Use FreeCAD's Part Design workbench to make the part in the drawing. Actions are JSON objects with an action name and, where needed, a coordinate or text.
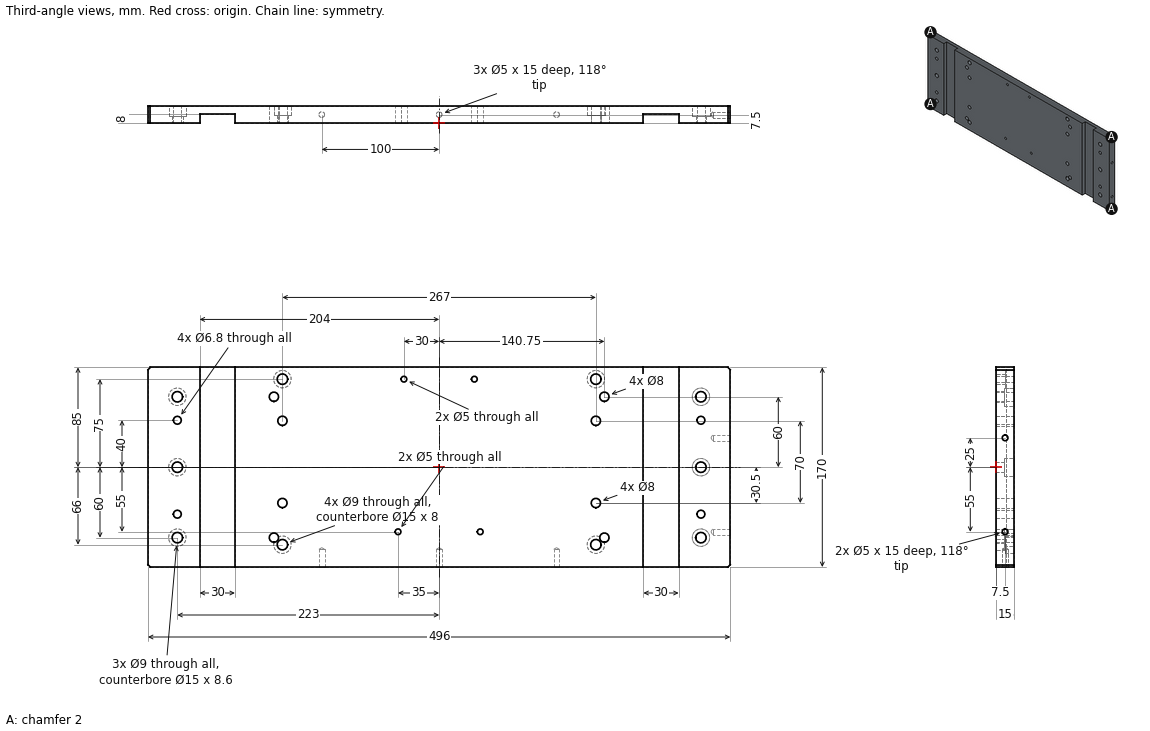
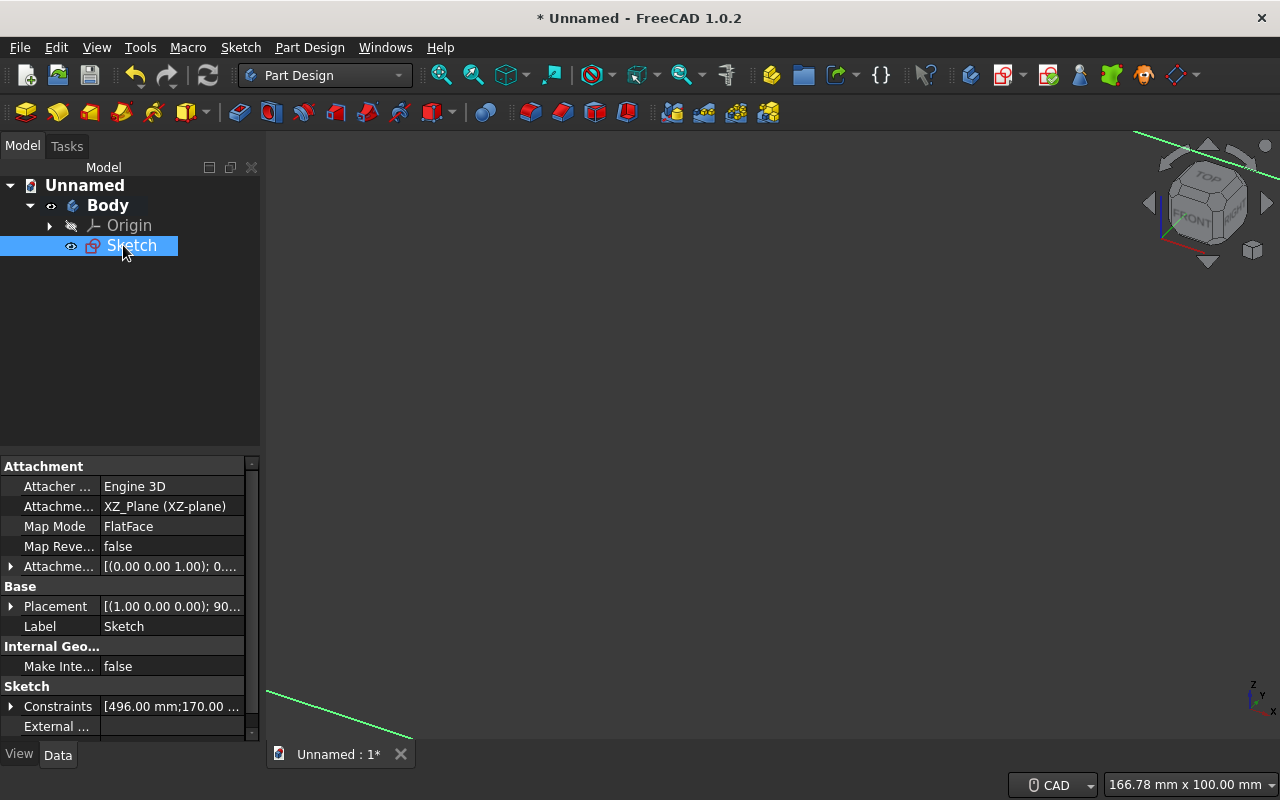
{"action": "left_click", "coordinate": [26, 112]}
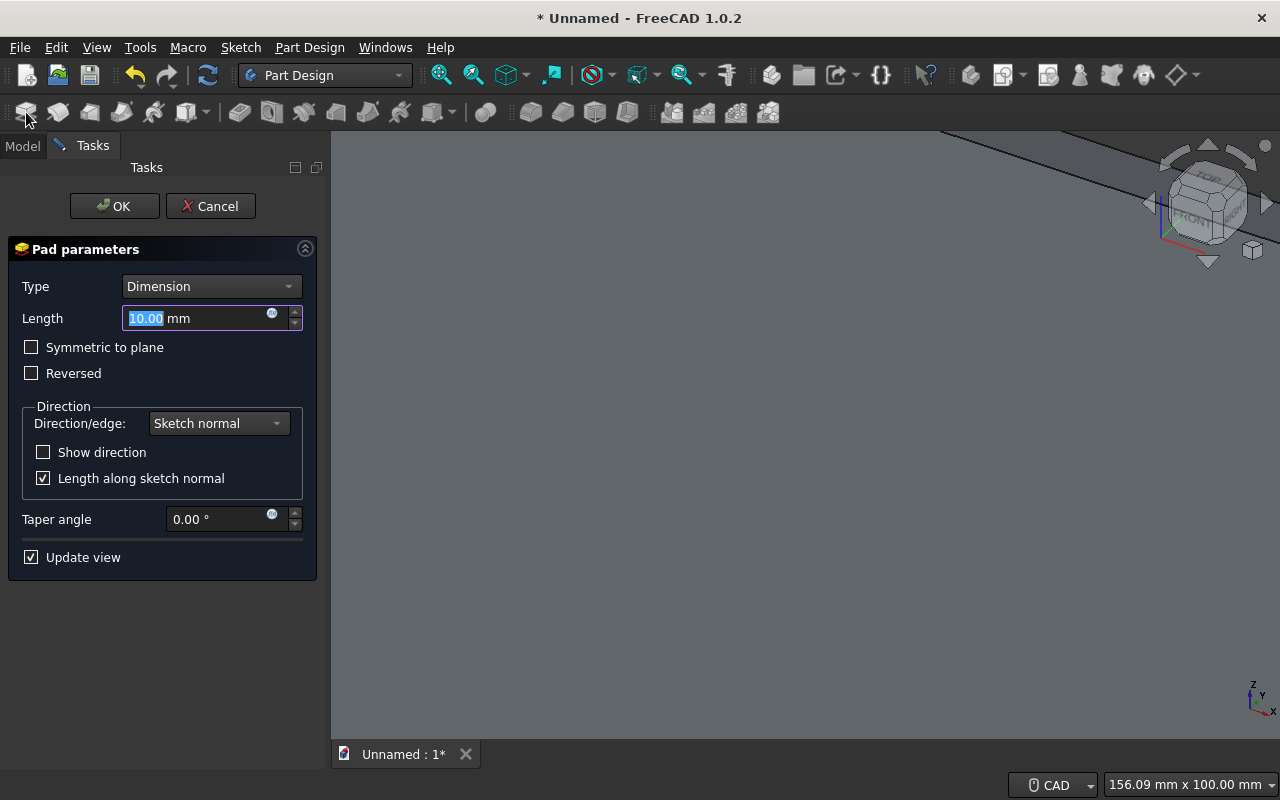
{"action": "type", "text": "15"}
{"action": "key", "text": "Tab"}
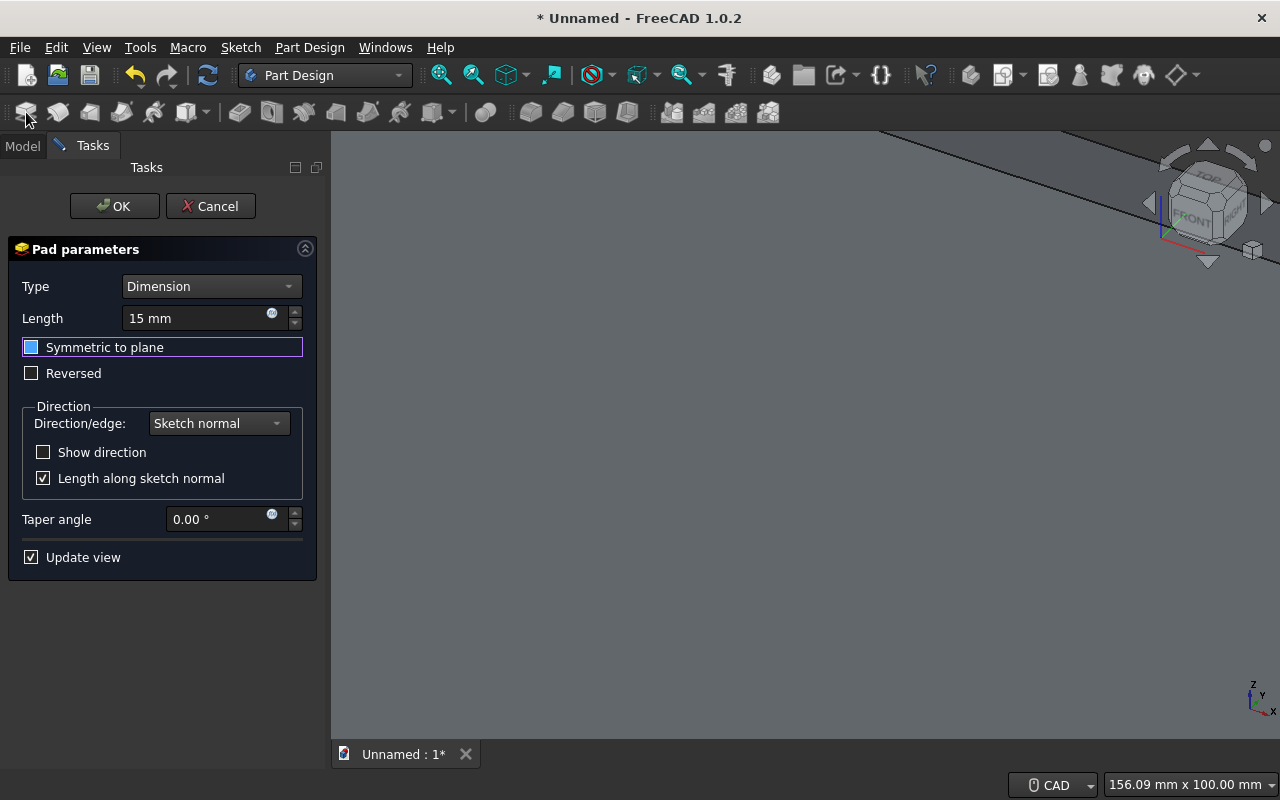
{"action": "left_click", "coordinate": [30, 373]}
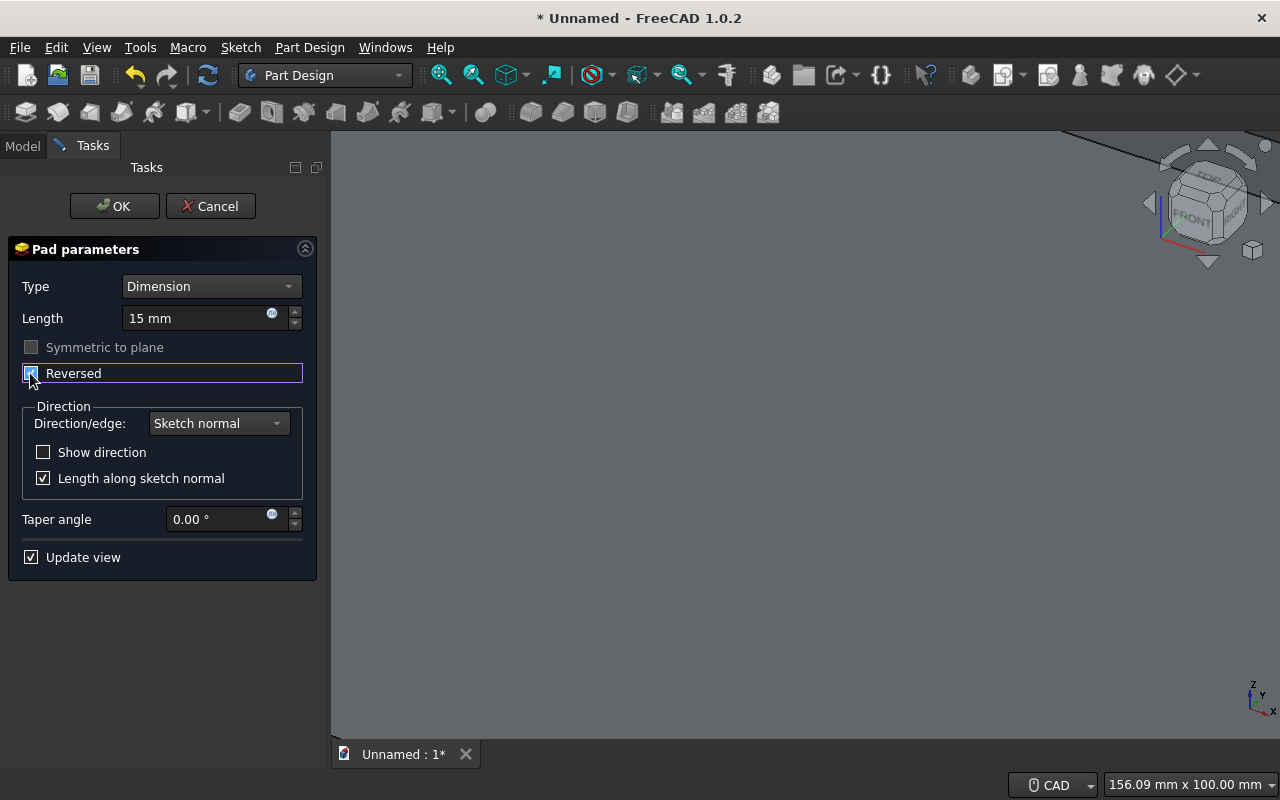
{"action": "left_click", "coordinate": [115, 206]}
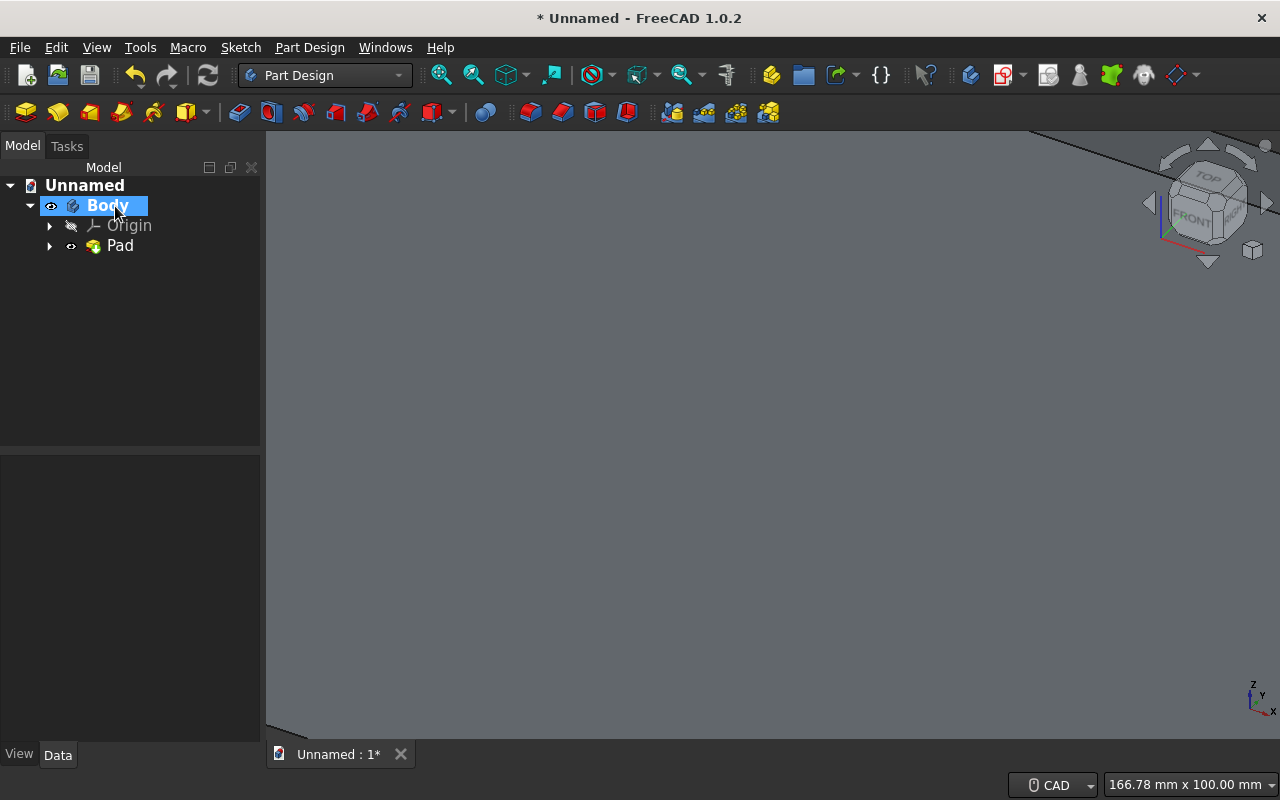
{"action": "left_click", "coordinate": [442, 76]}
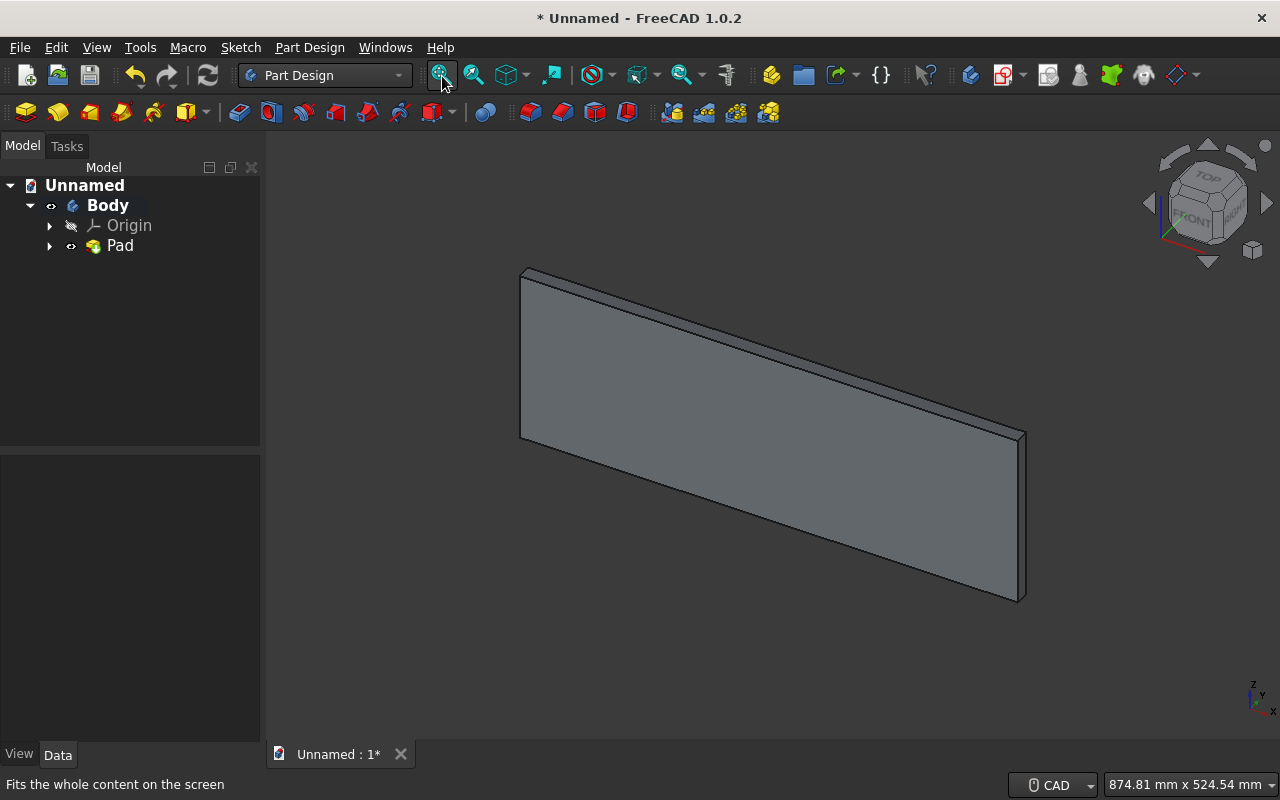
{"action": "key", "text": "4"}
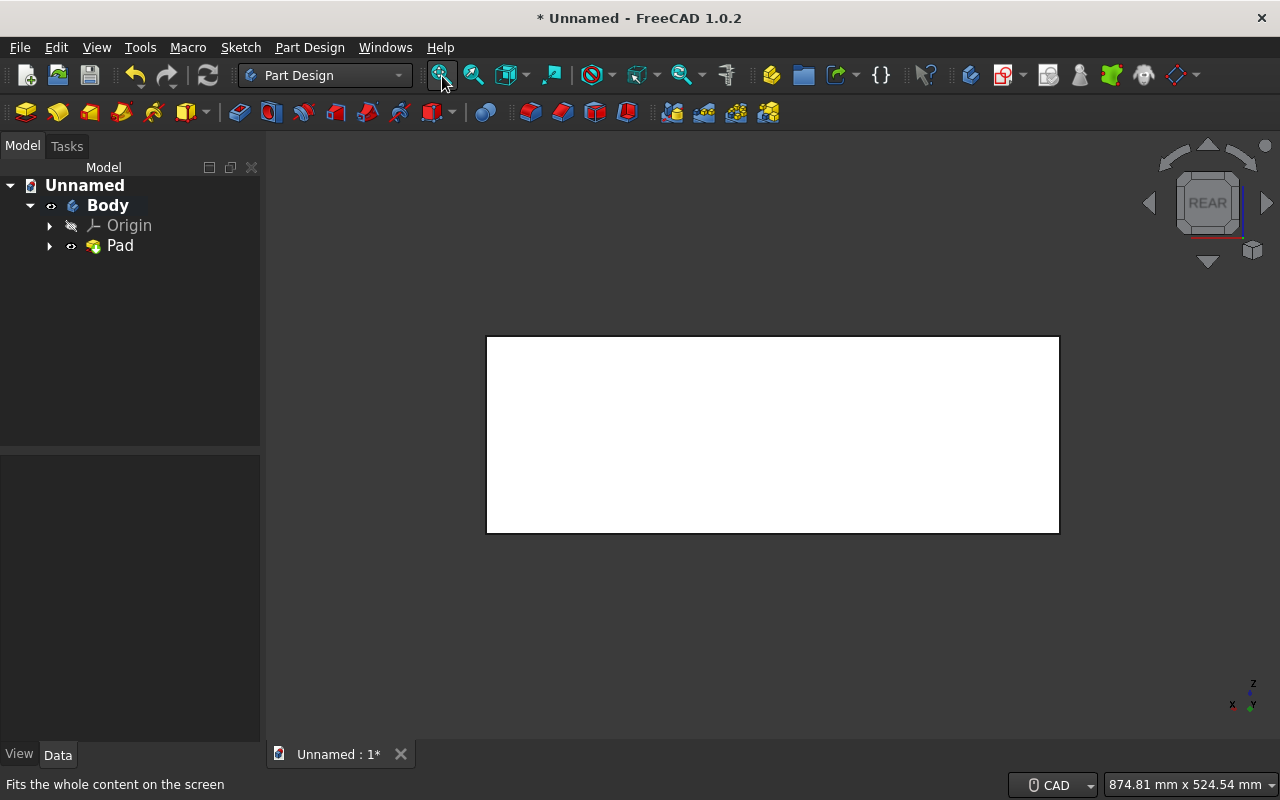
{"action": "left_click", "coordinate": [609, 434]}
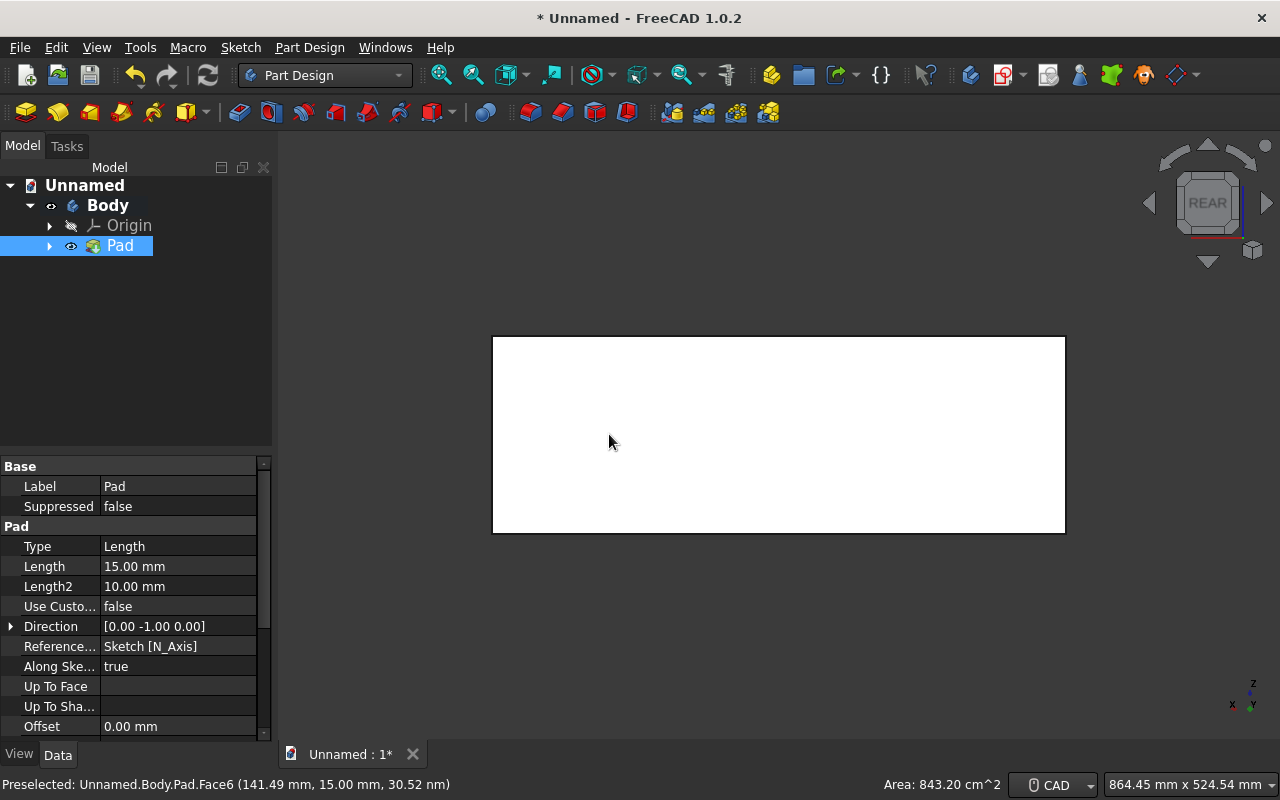
{"action": "left_click", "coordinate": [1004, 76]}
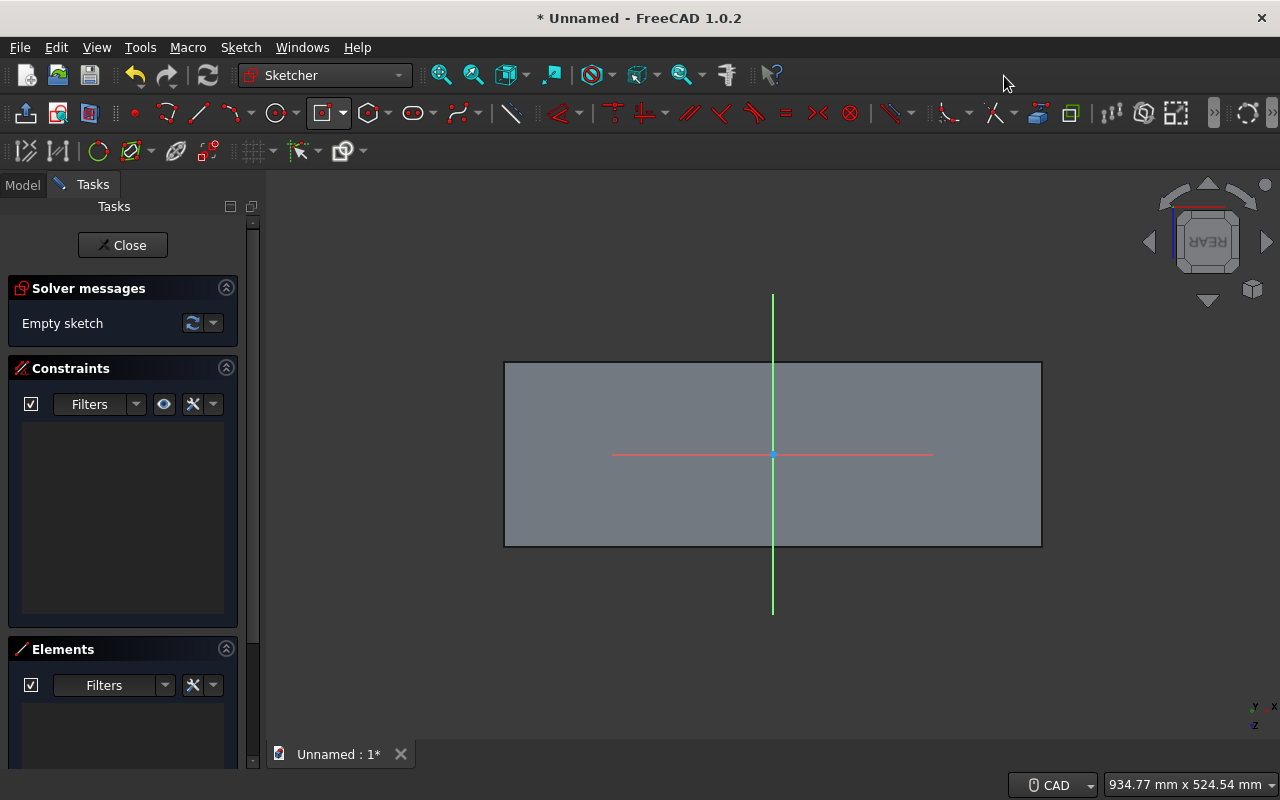
{"action": "scroll", "coordinate": [605, 454], "scroll_direction": "up", "scroll_amount": 4}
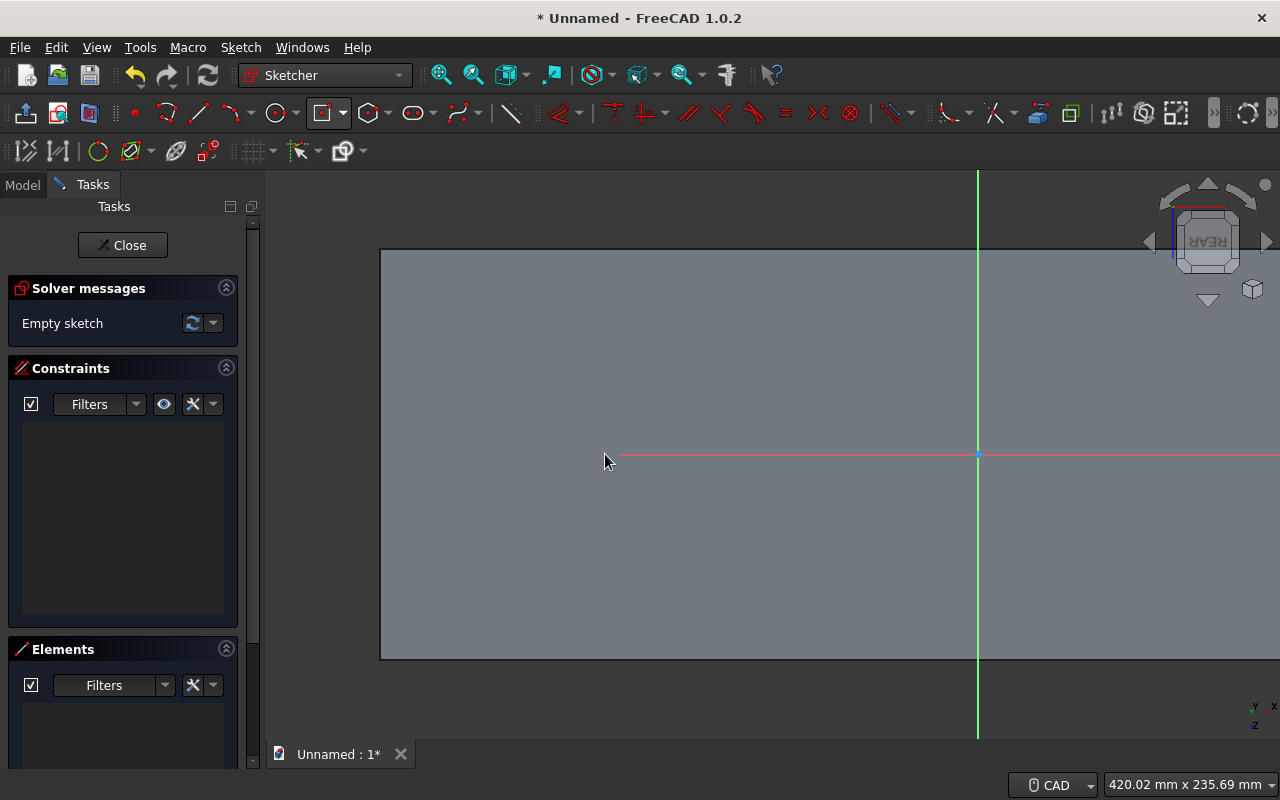
{"action": "left_click", "coordinate": [276, 114]}